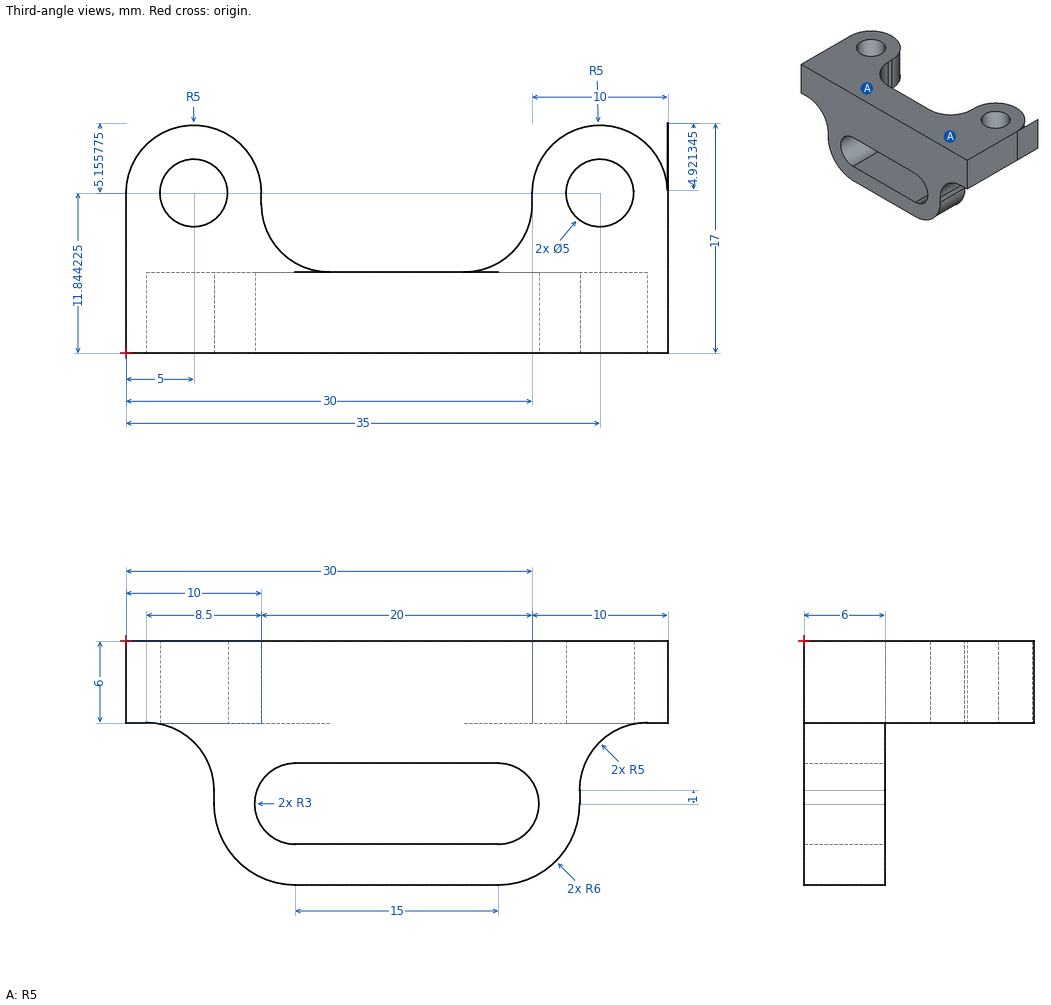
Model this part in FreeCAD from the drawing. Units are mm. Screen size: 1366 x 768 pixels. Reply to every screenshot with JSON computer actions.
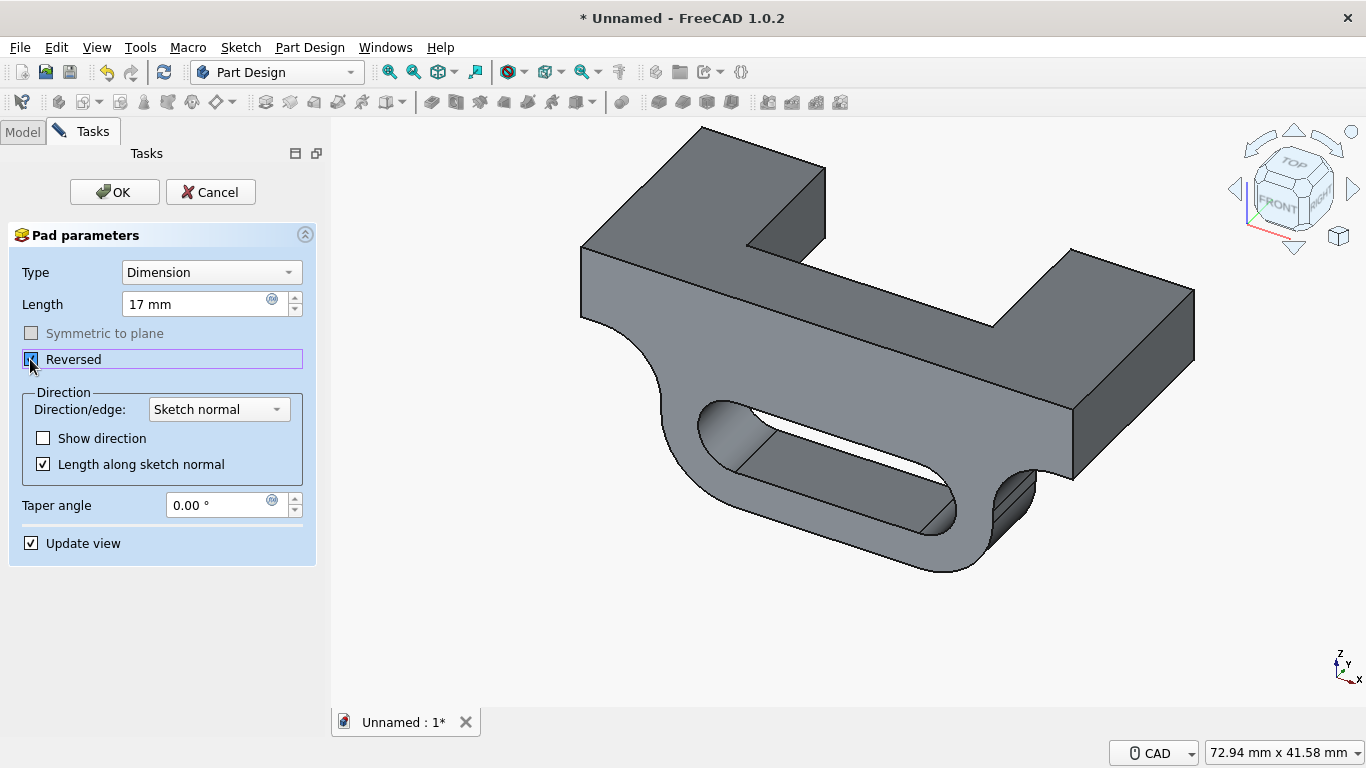
{"action": "left_click", "coordinate": [115, 192]}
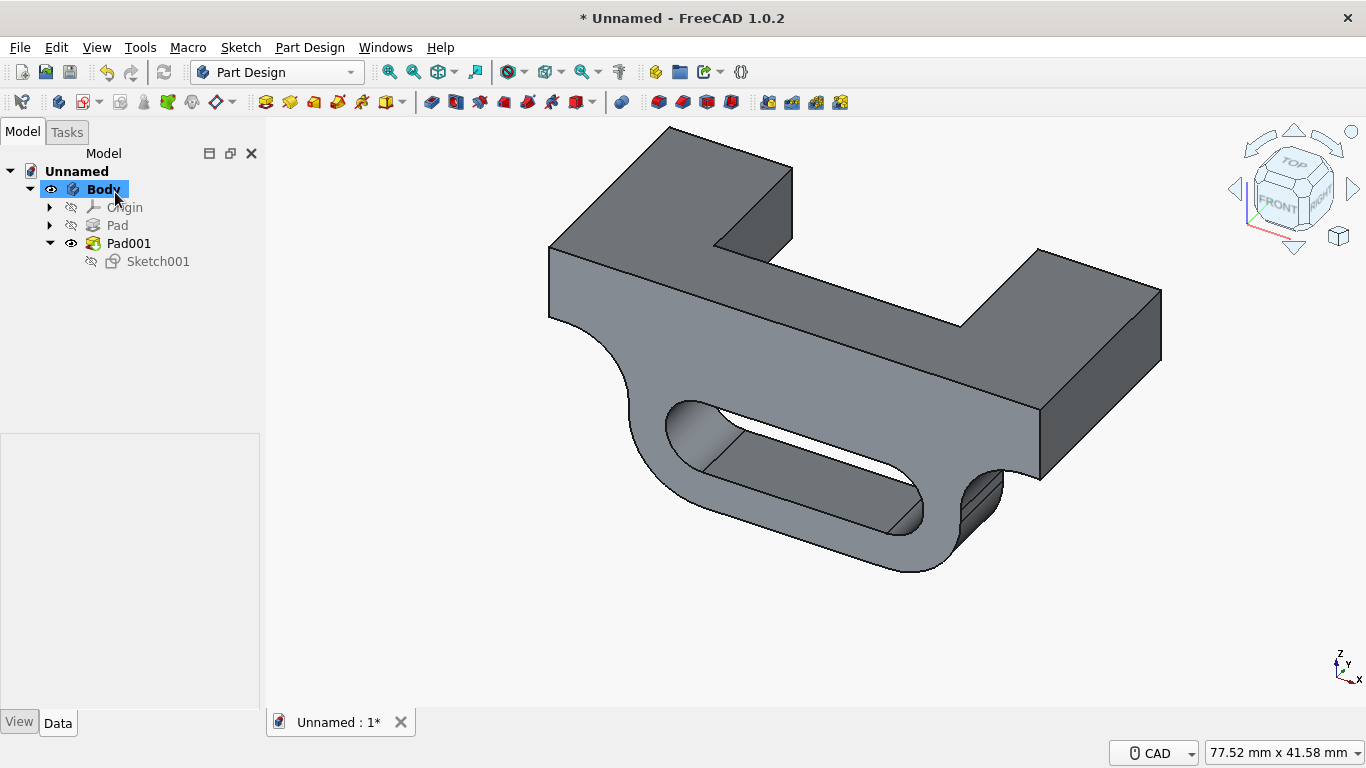
{"action": "key", "text": "0"}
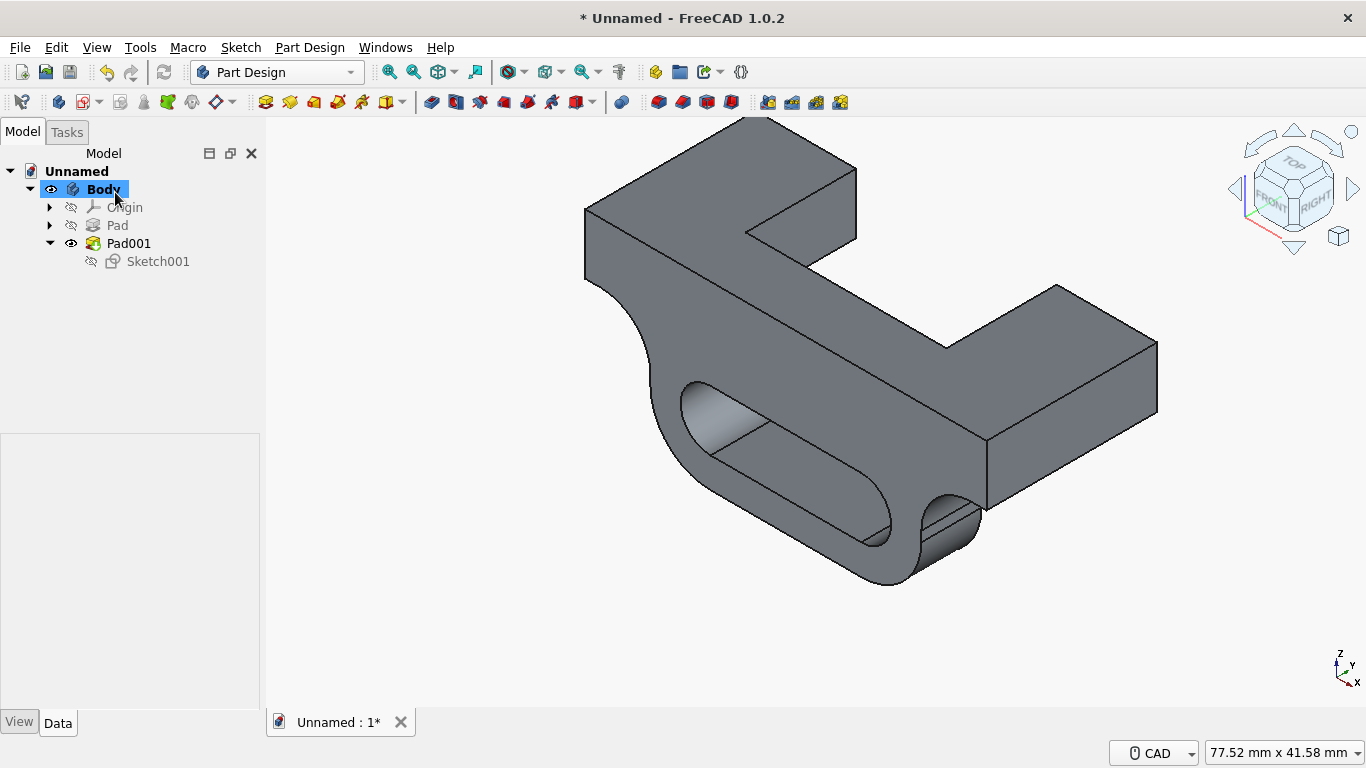
{"action": "key", "text": "v f"}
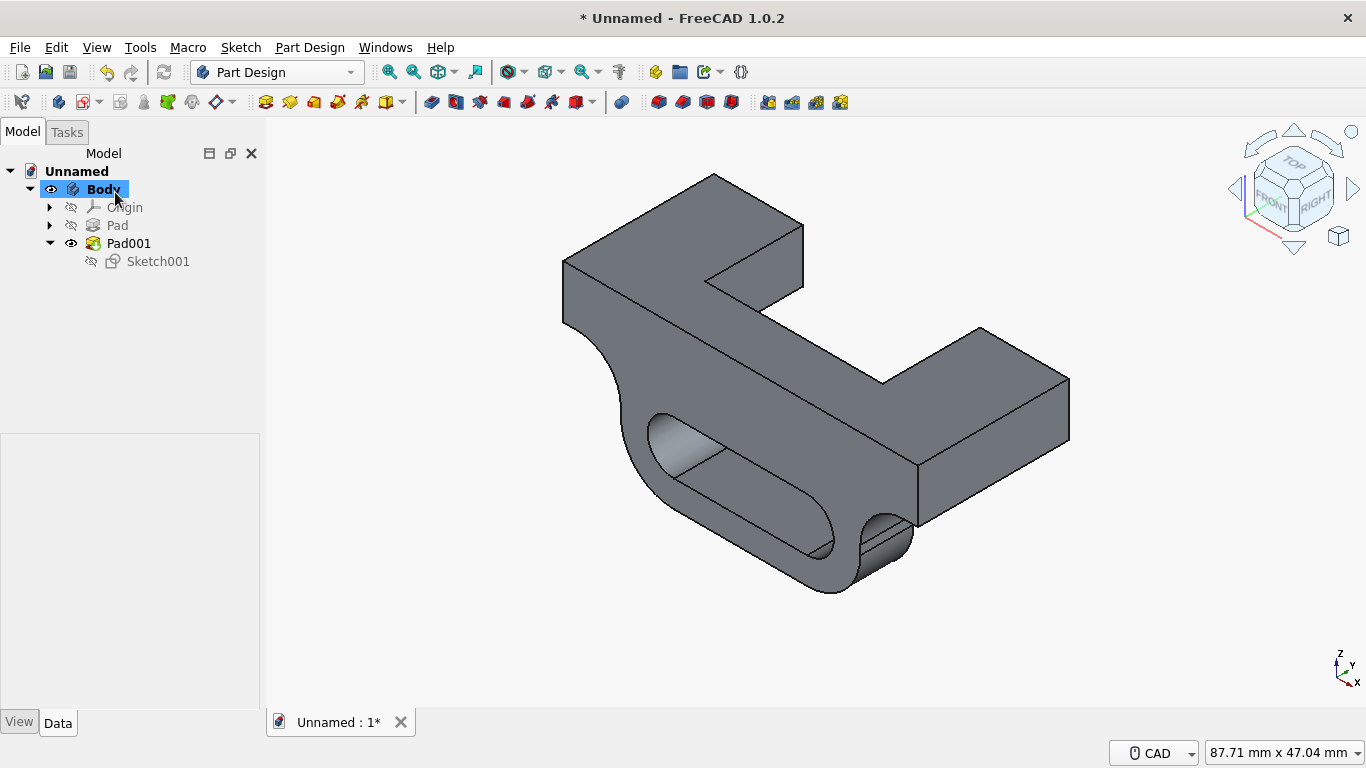
{"action": "key", "text": "2"}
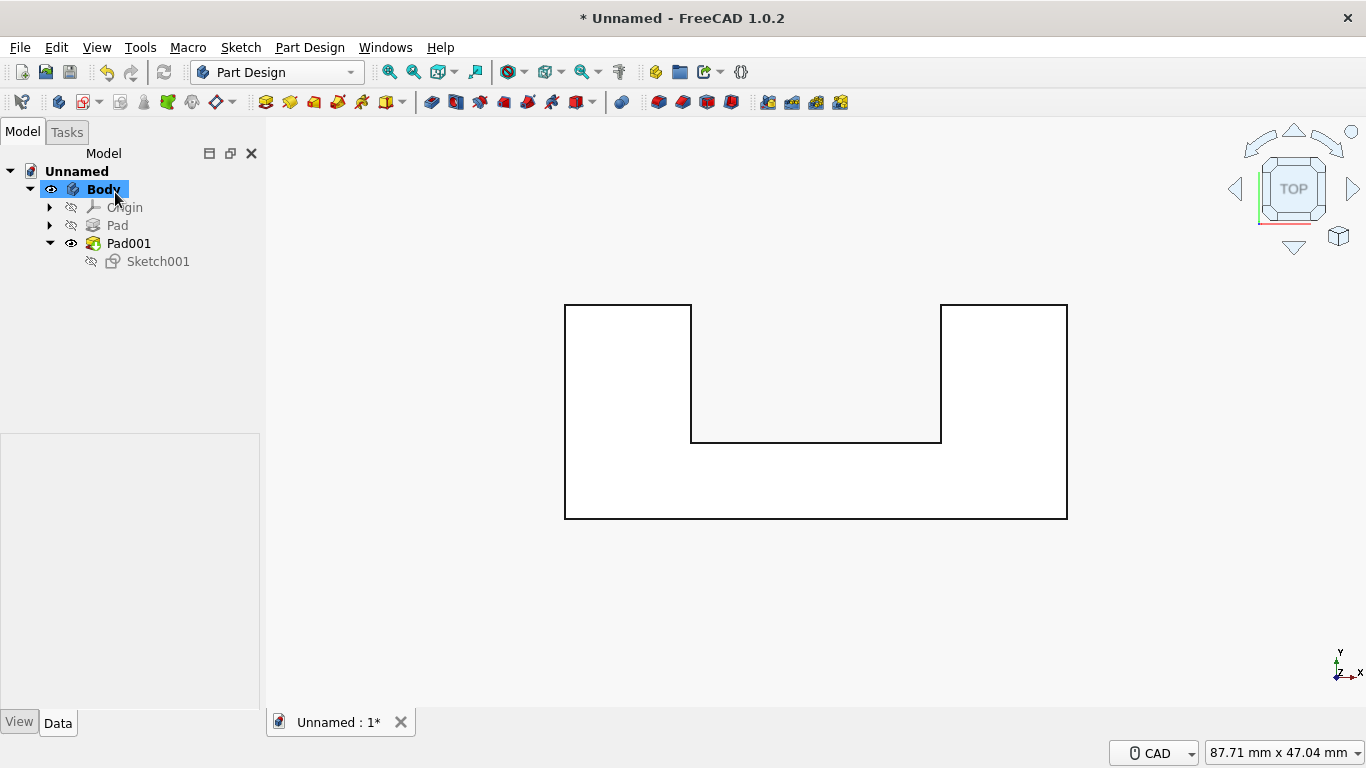
{"action": "key", "text": "1"}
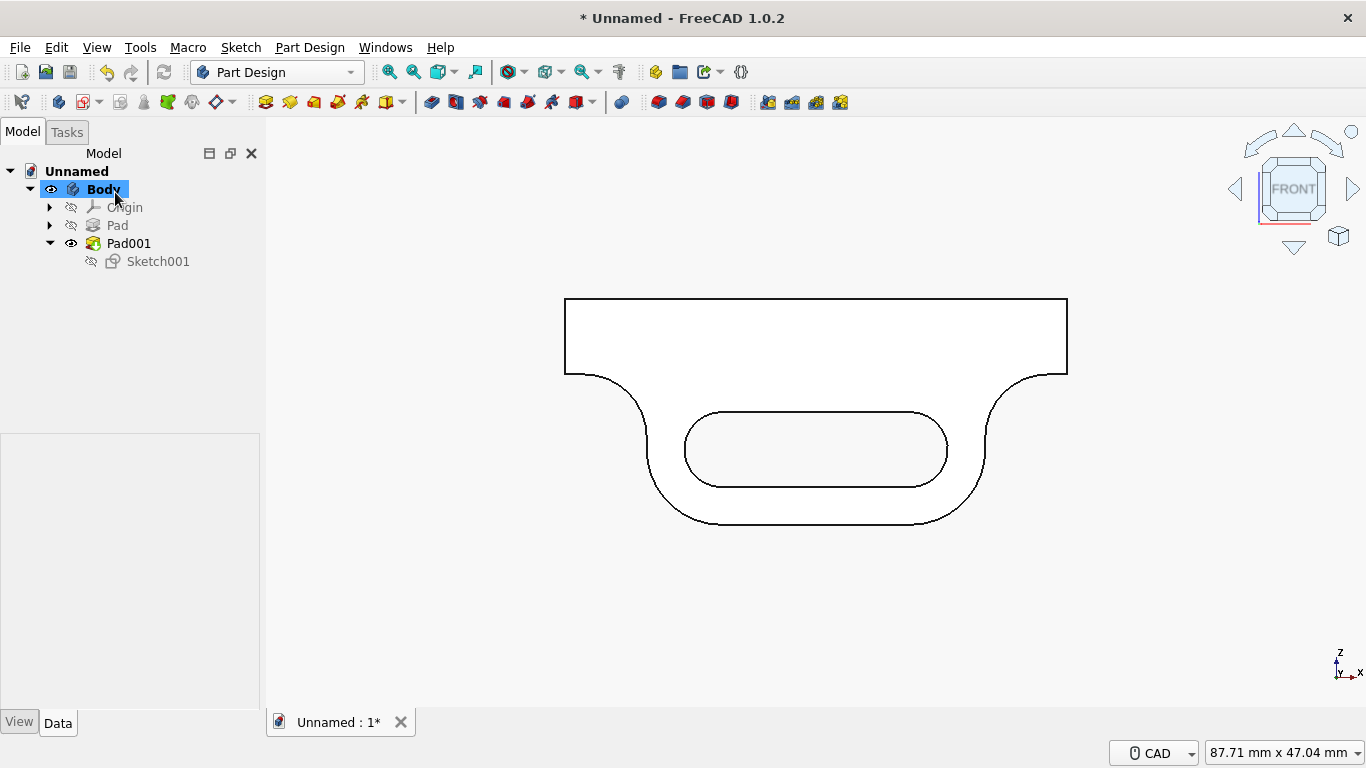
{"action": "key", "text": "3"}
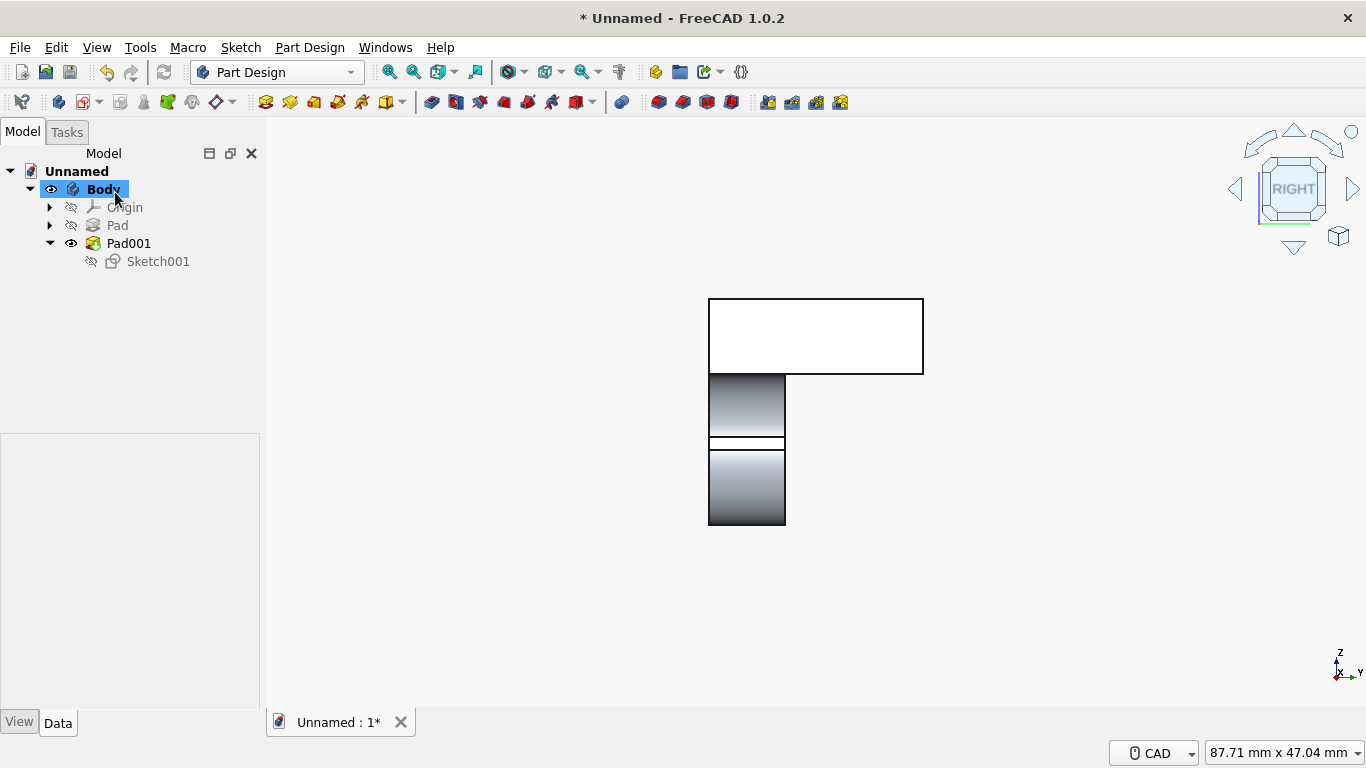
{"action": "left_click", "coordinate": [390, 72]}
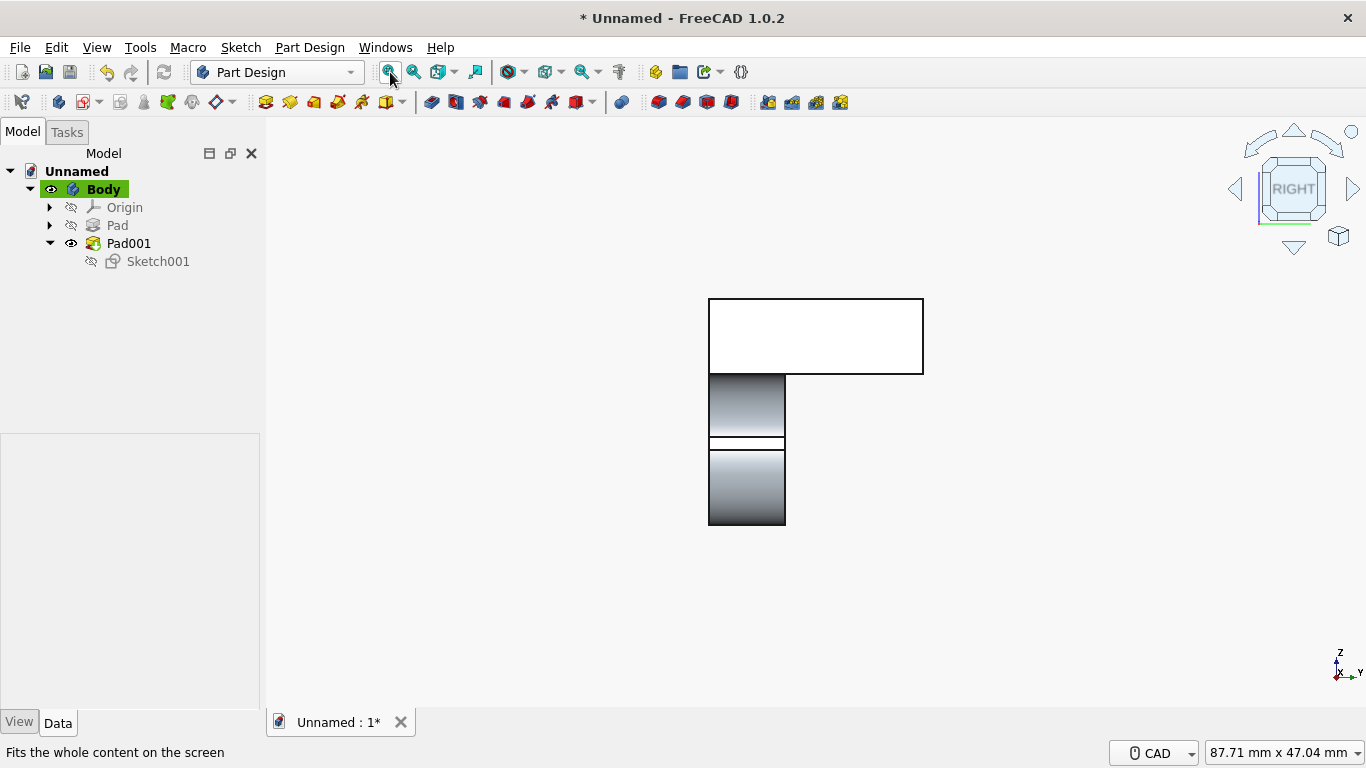
{"action": "key", "text": "5"}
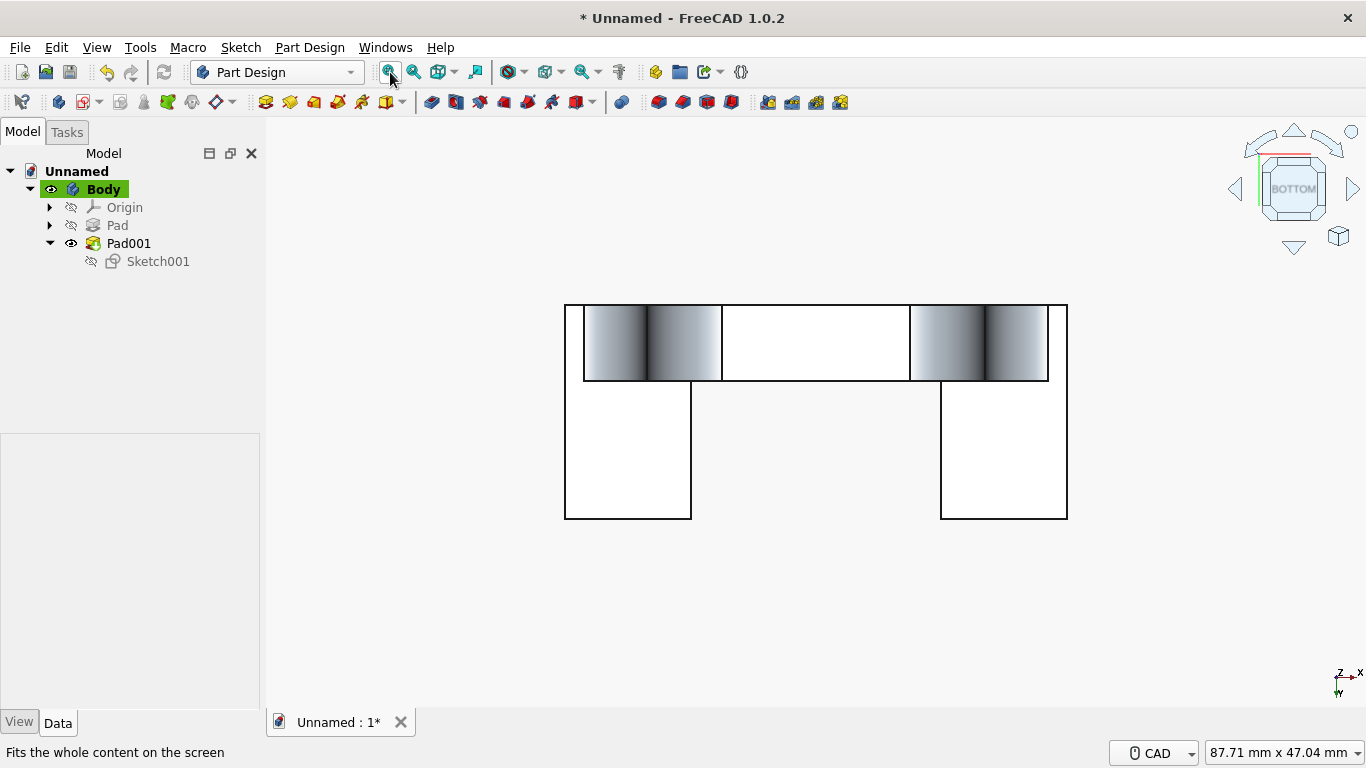
{"action": "key", "text": "4"}